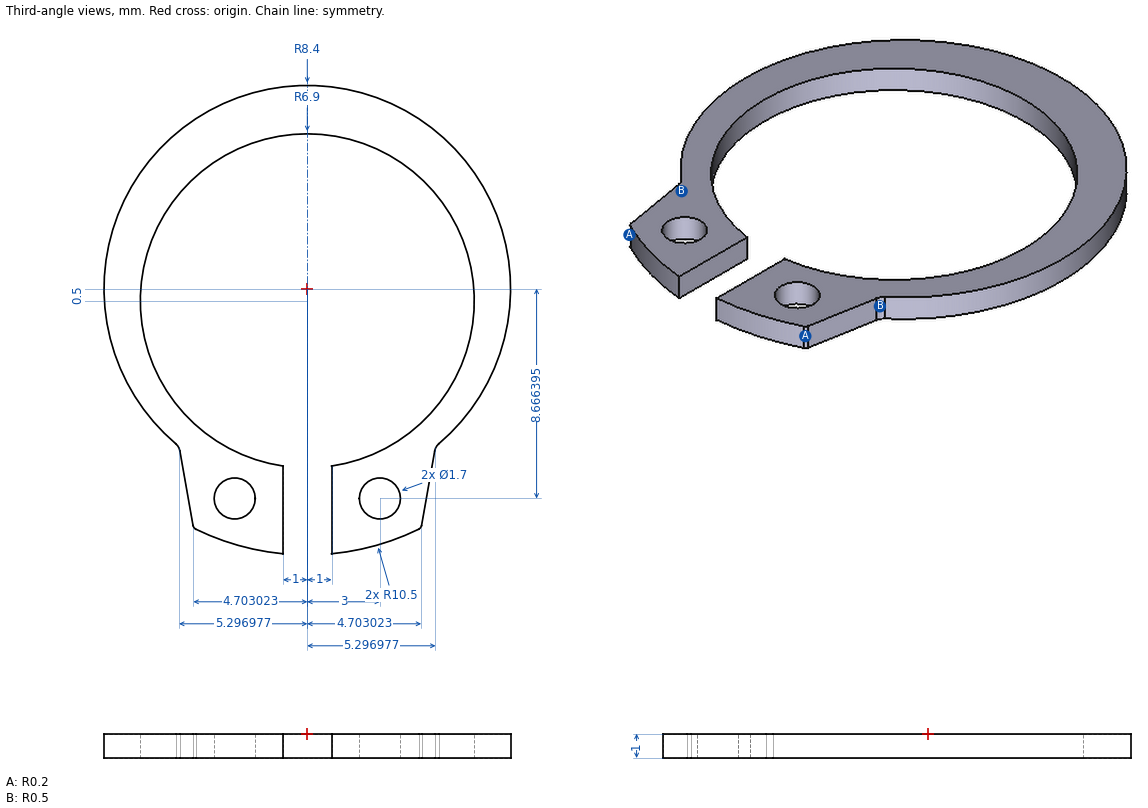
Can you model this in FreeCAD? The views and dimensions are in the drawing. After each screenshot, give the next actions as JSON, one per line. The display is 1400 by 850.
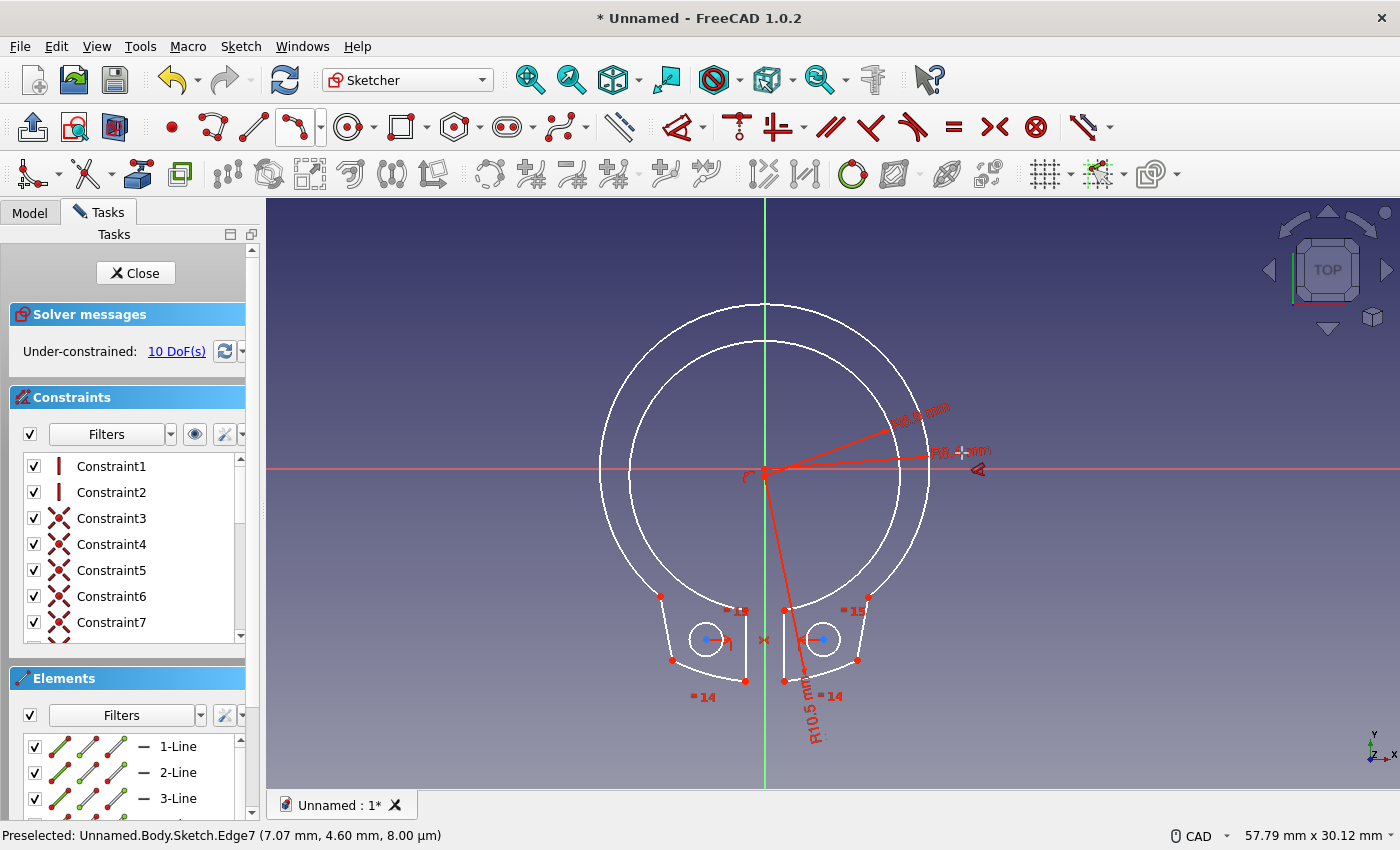
{"action": "left_click", "coordinate": [835, 628]}
{"action": "left_click", "coordinate": [892, 620]}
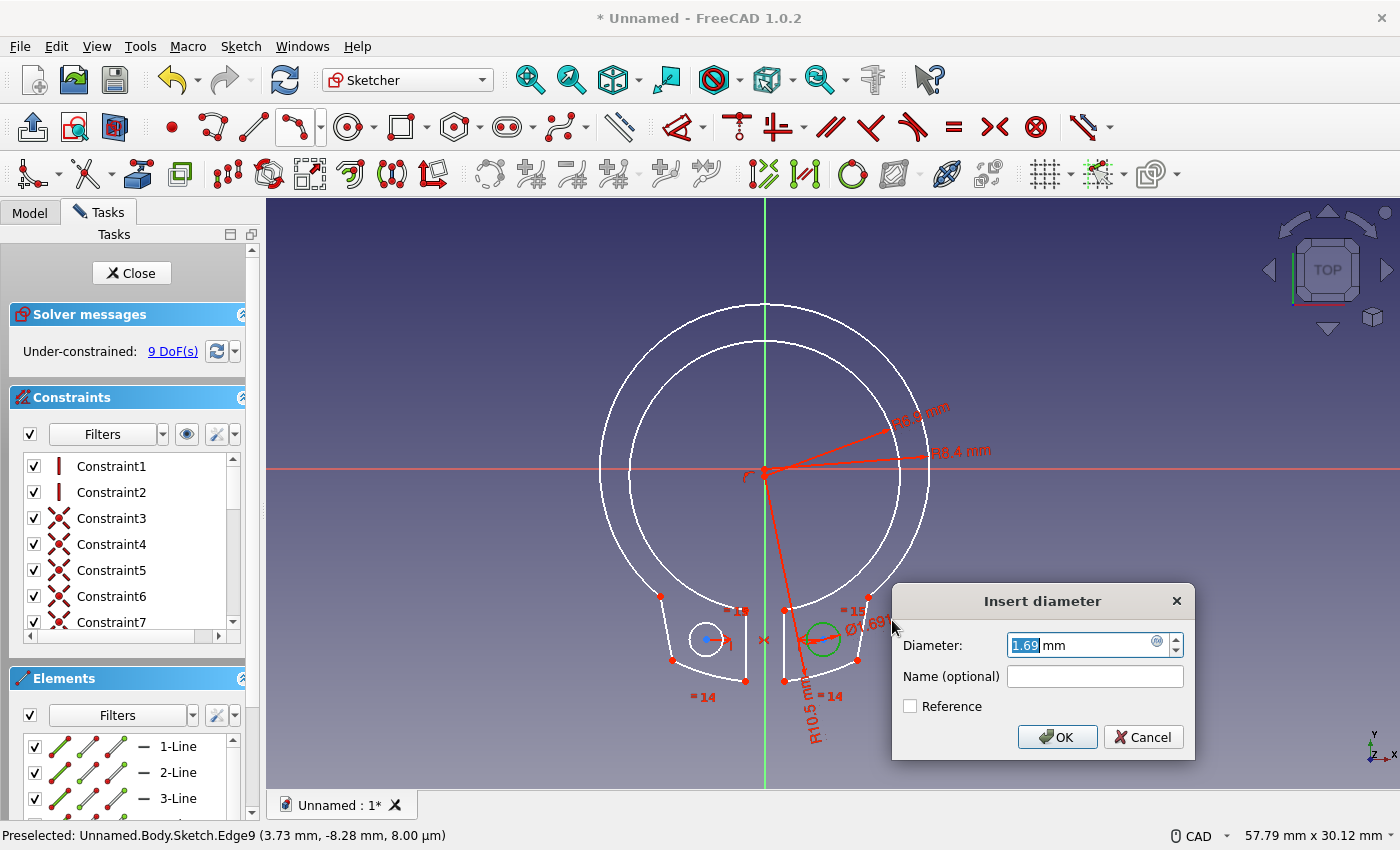
{"action": "type", "text": "1.7"}
{"action": "key", "text": "Return"}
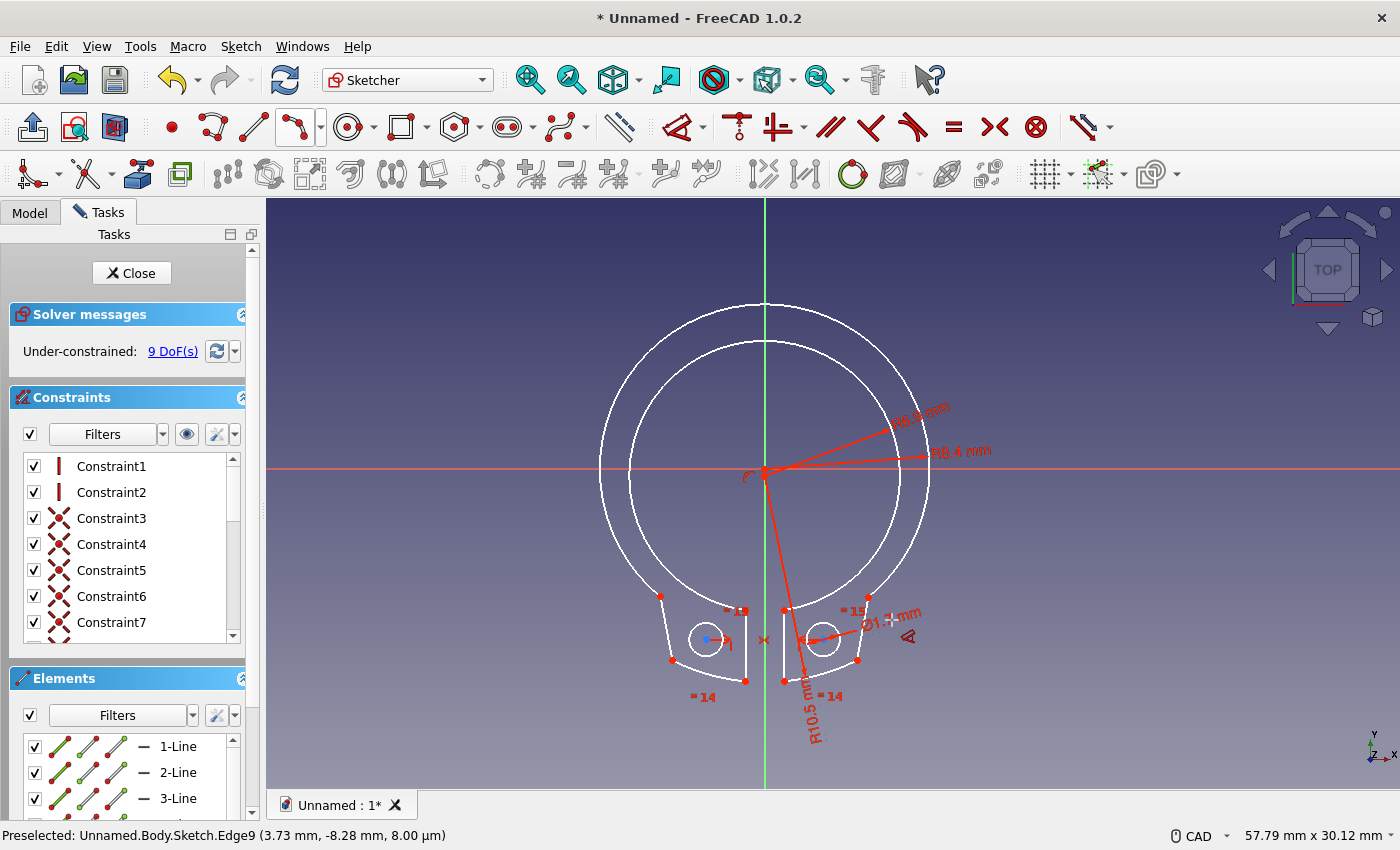
{"action": "left_click", "coordinate": [823, 640]}
{"action": "left_click", "coordinate": [794, 435]}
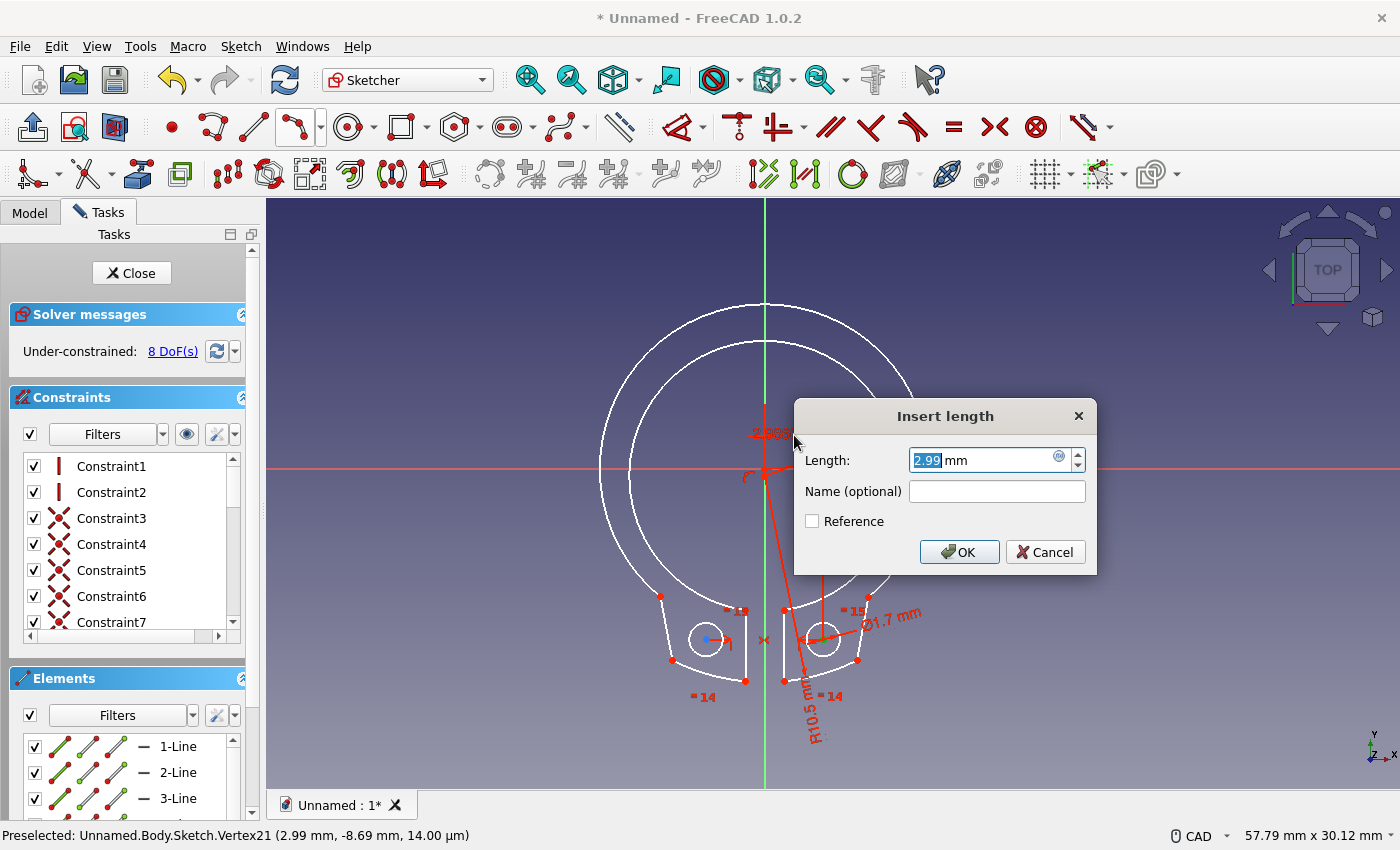
{"action": "type", "text": "3"}
{"action": "key", "text": "Return"}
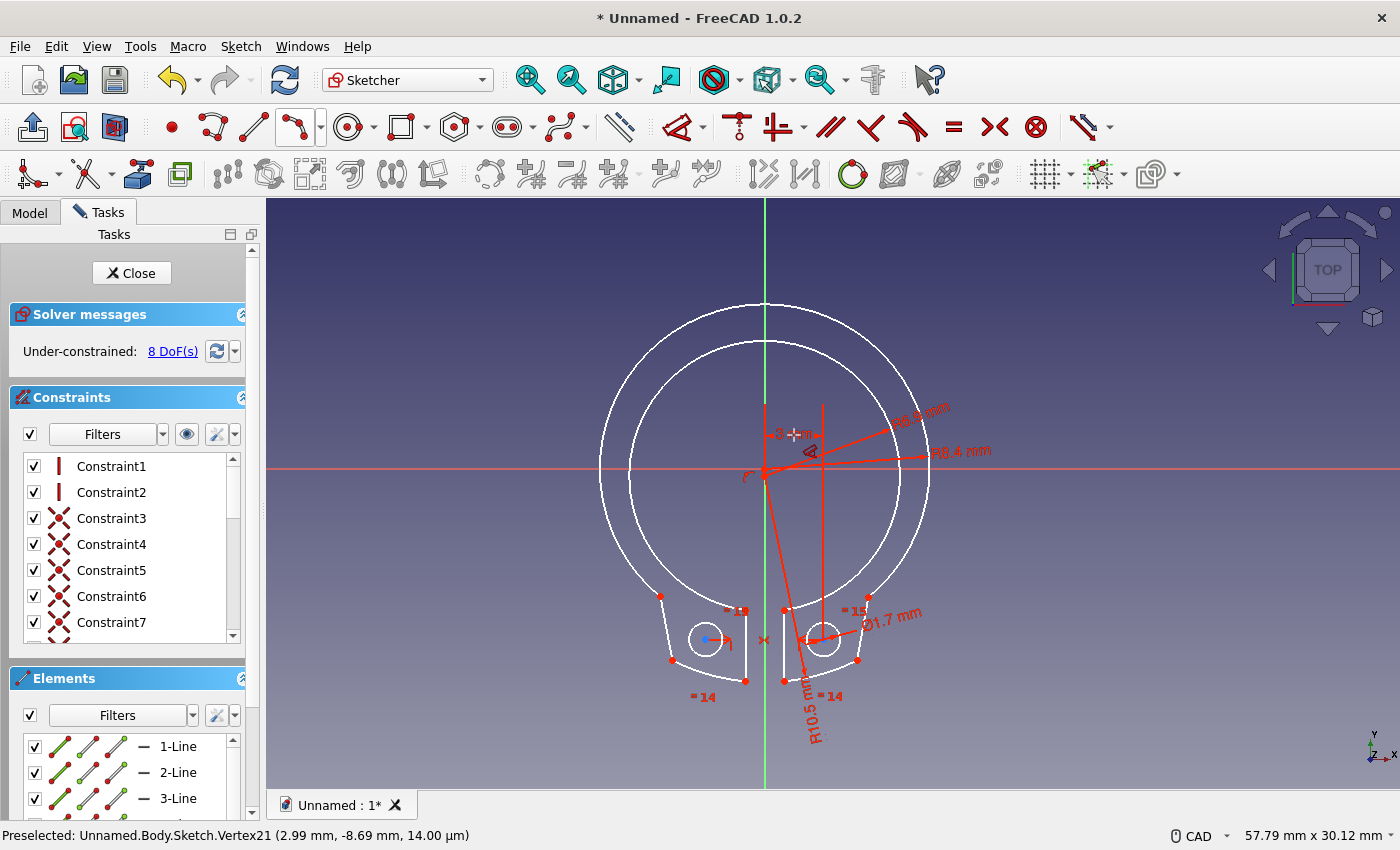
{"action": "scroll", "coordinate": [746, 681], "scroll_direction": "up", "scroll_amount": 4}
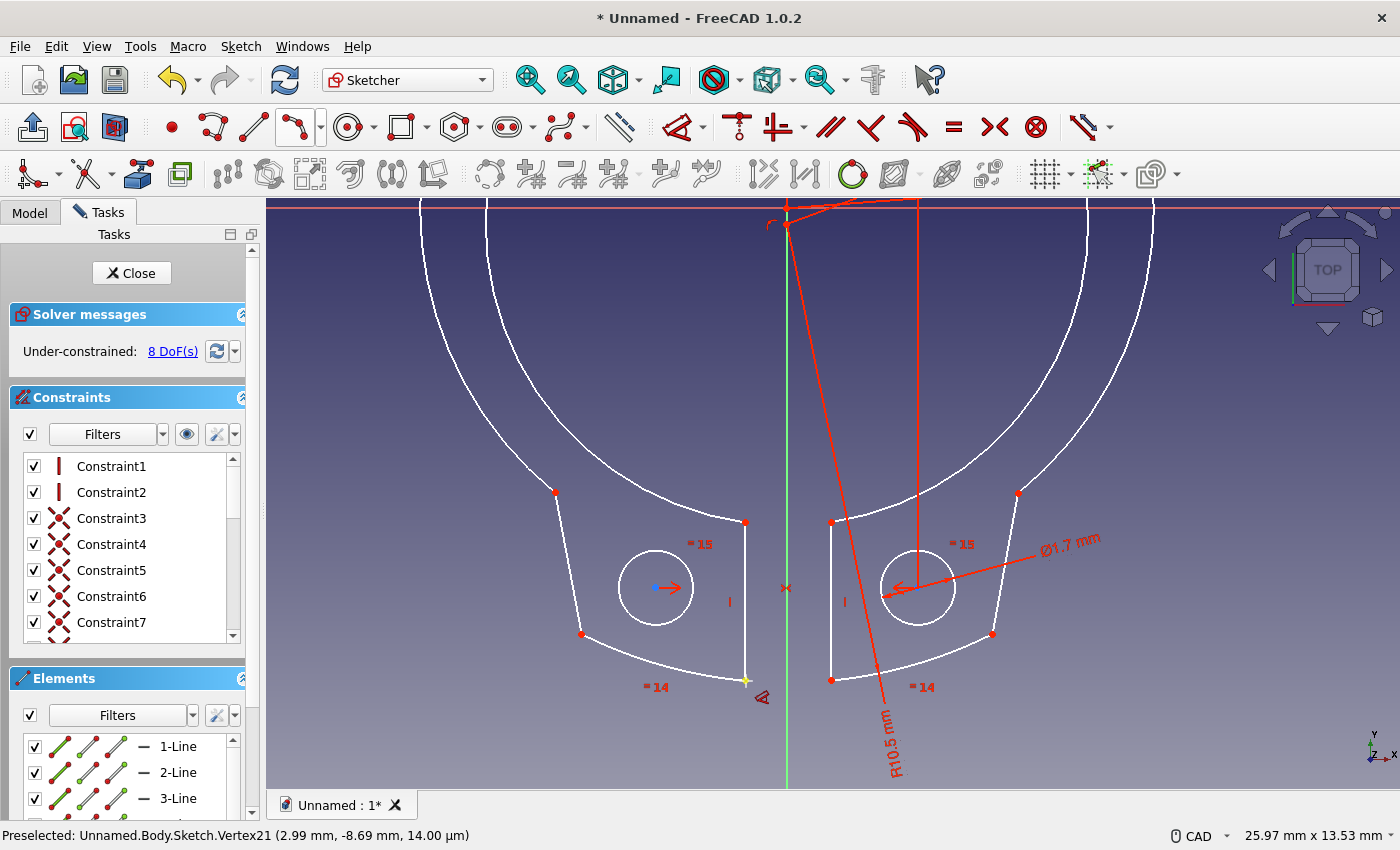
{"action": "left_click", "coordinate": [745, 681]}
{"action": "left_click", "coordinate": [766, 715]}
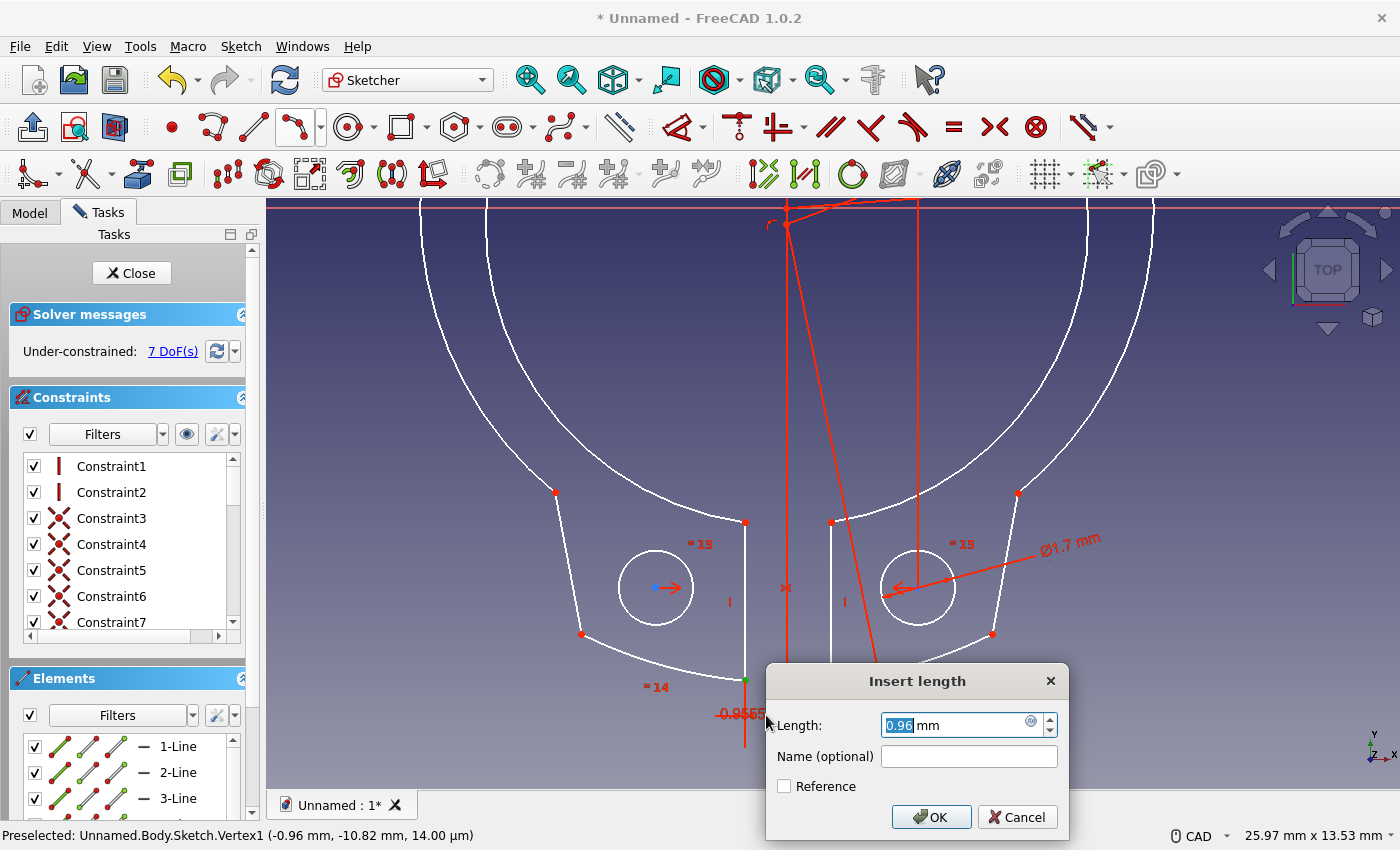
{"action": "type", "text": "1"}
{"action": "key", "text": "Return"}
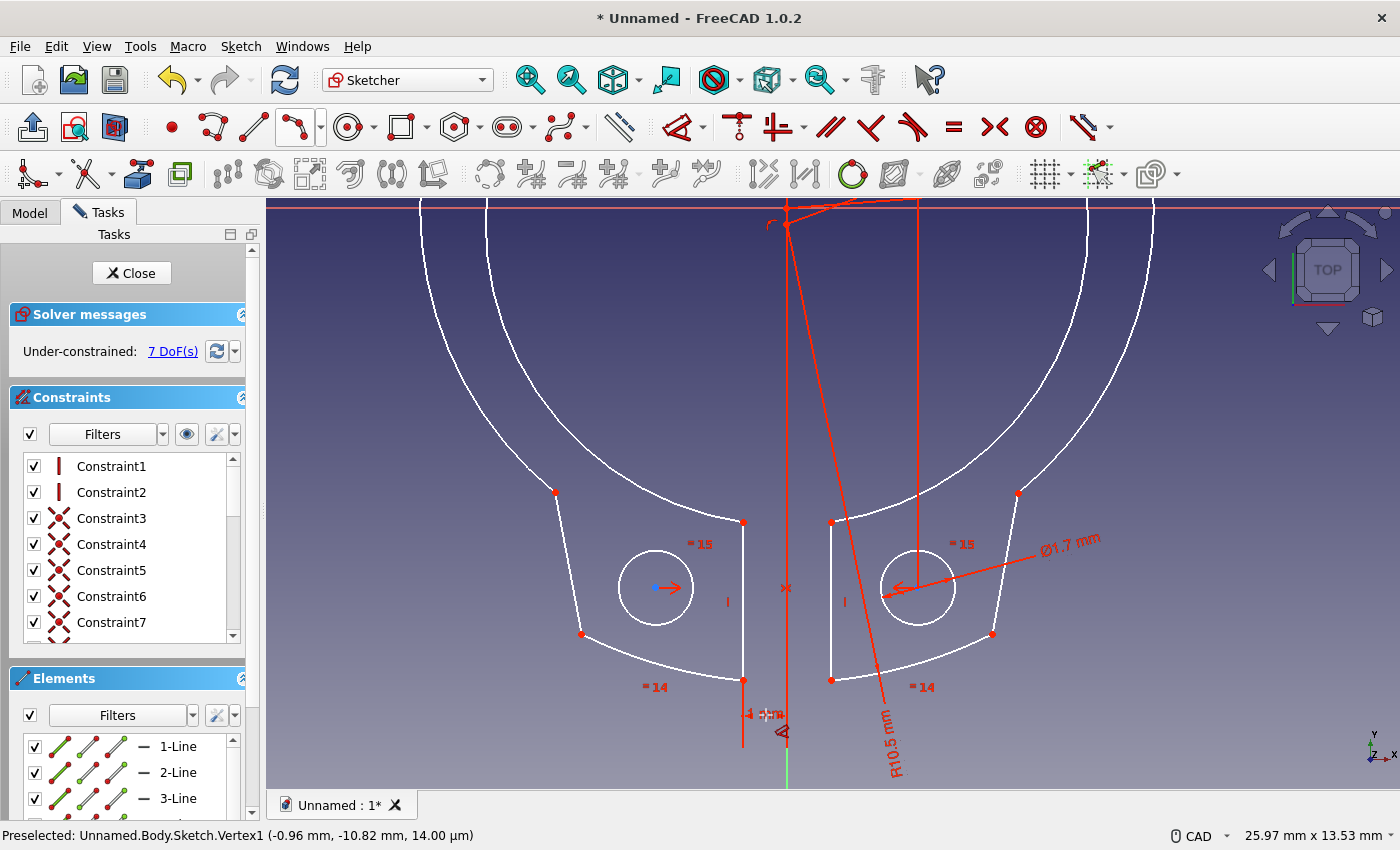
{"action": "left_click", "coordinate": [831, 522]}
{"action": "left_click", "coordinate": [809, 556]}